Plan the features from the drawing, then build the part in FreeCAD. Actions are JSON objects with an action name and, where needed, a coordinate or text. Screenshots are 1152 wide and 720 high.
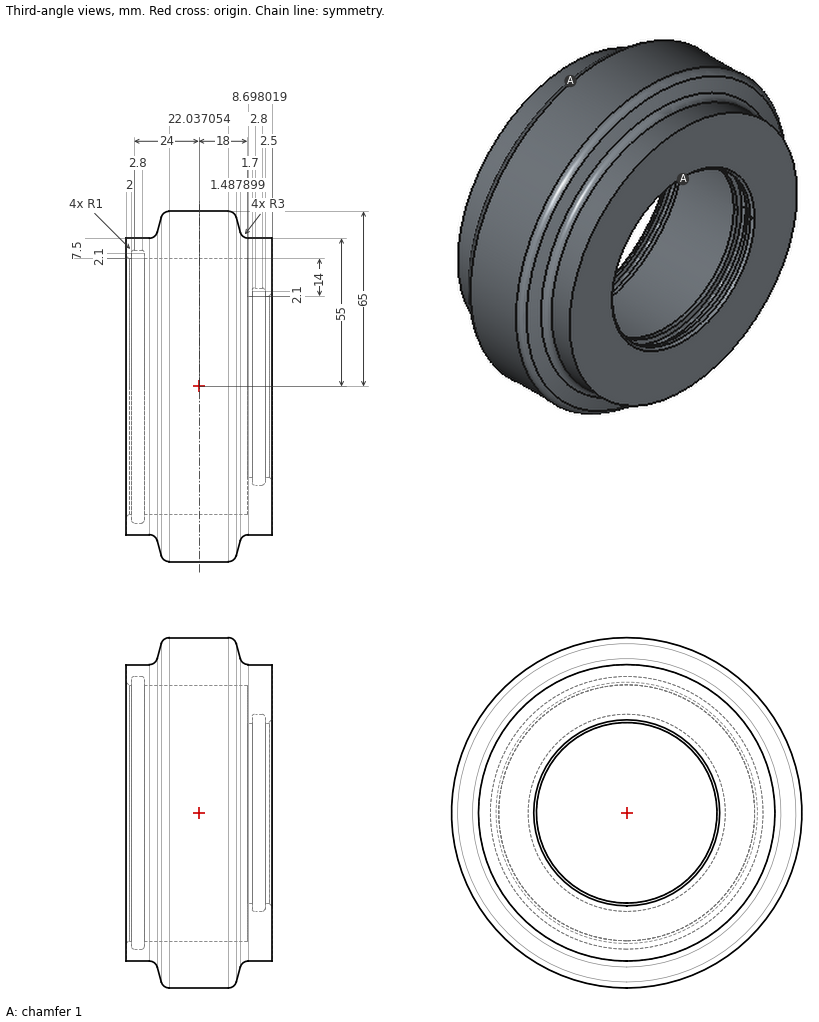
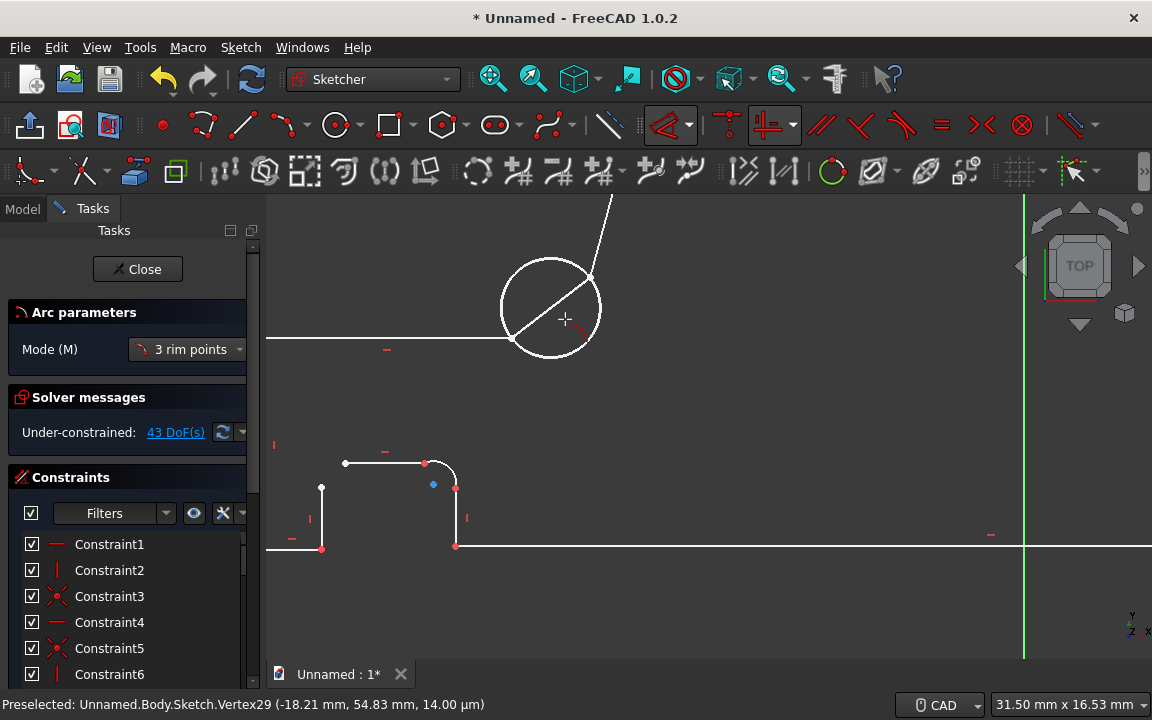
{"action": "left_click", "coordinate": [560, 316]}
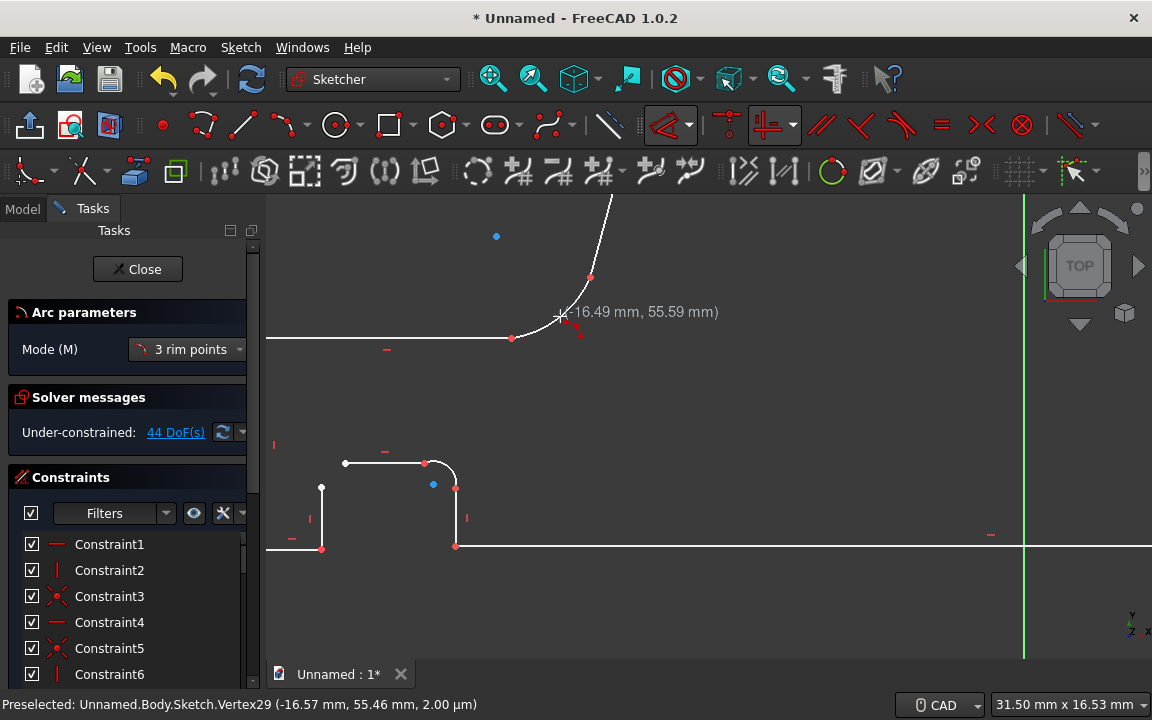
{"action": "left_click", "coordinate": [322, 488]}
{"action": "left_click", "coordinate": [346, 463]}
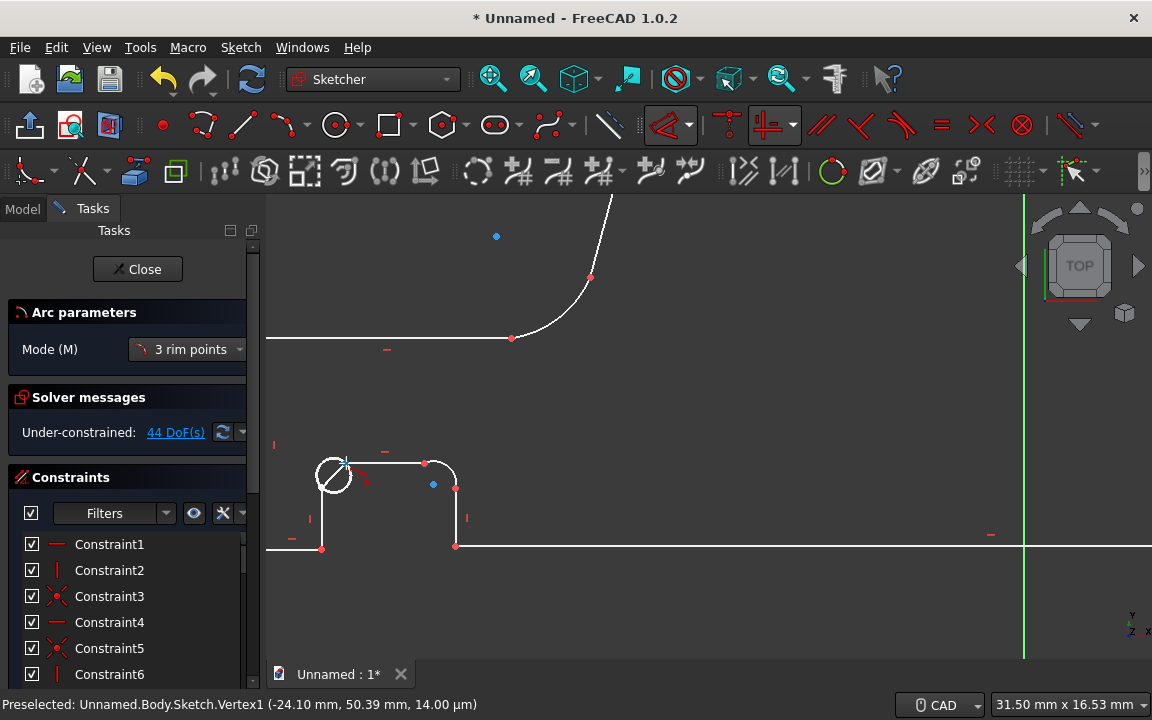
{"action": "scroll", "coordinate": [329, 465], "scroll_direction": "up", "scroll_amount": 4}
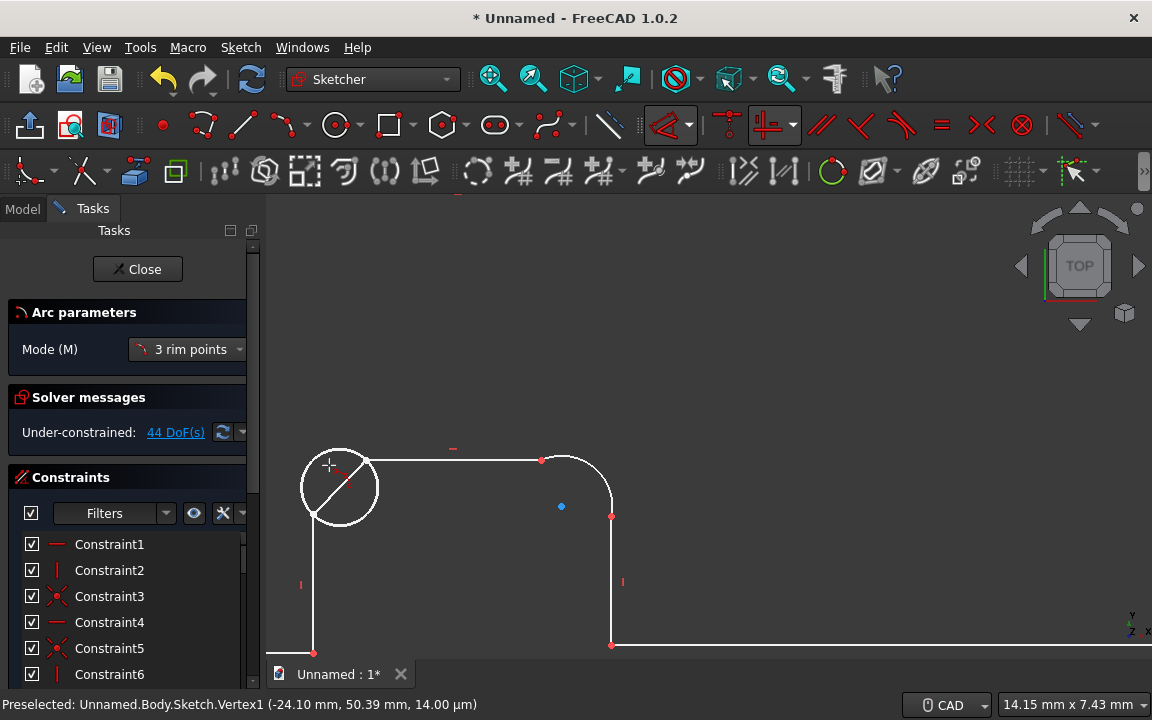
{"action": "left_click", "coordinate": [328, 465]}
{"action": "key", "text": "Escape"}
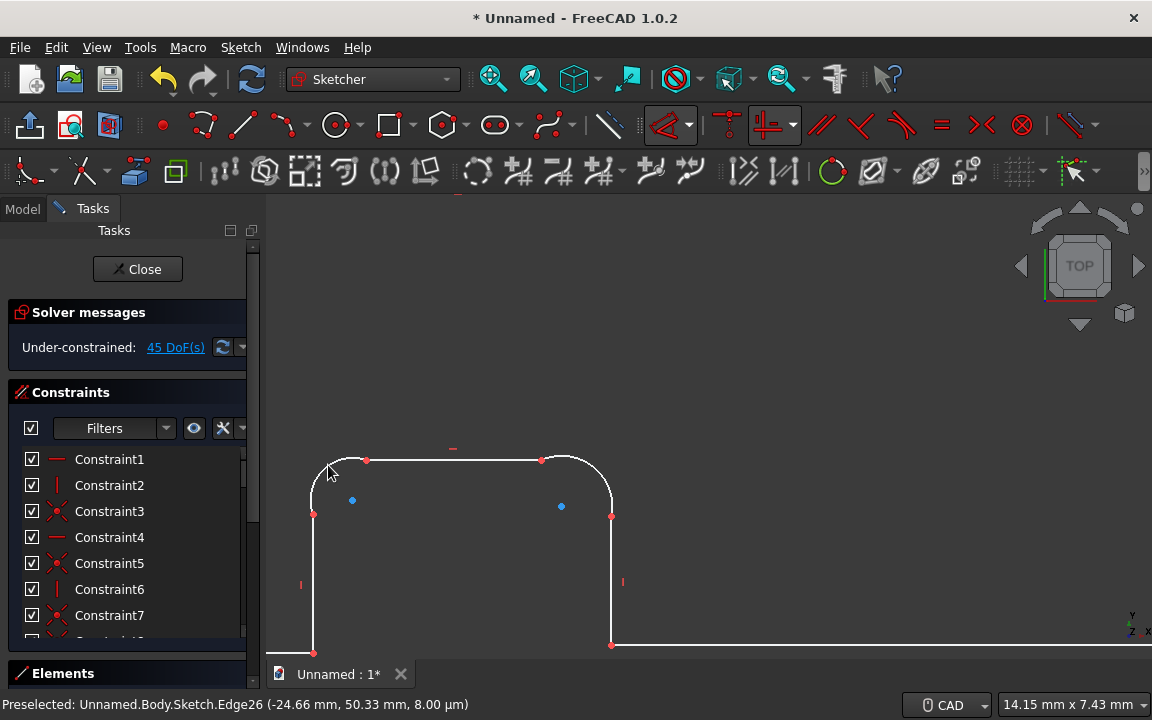
{"action": "scroll", "coordinate": [541, 334], "scroll_direction": "down", "scroll_amount": 13}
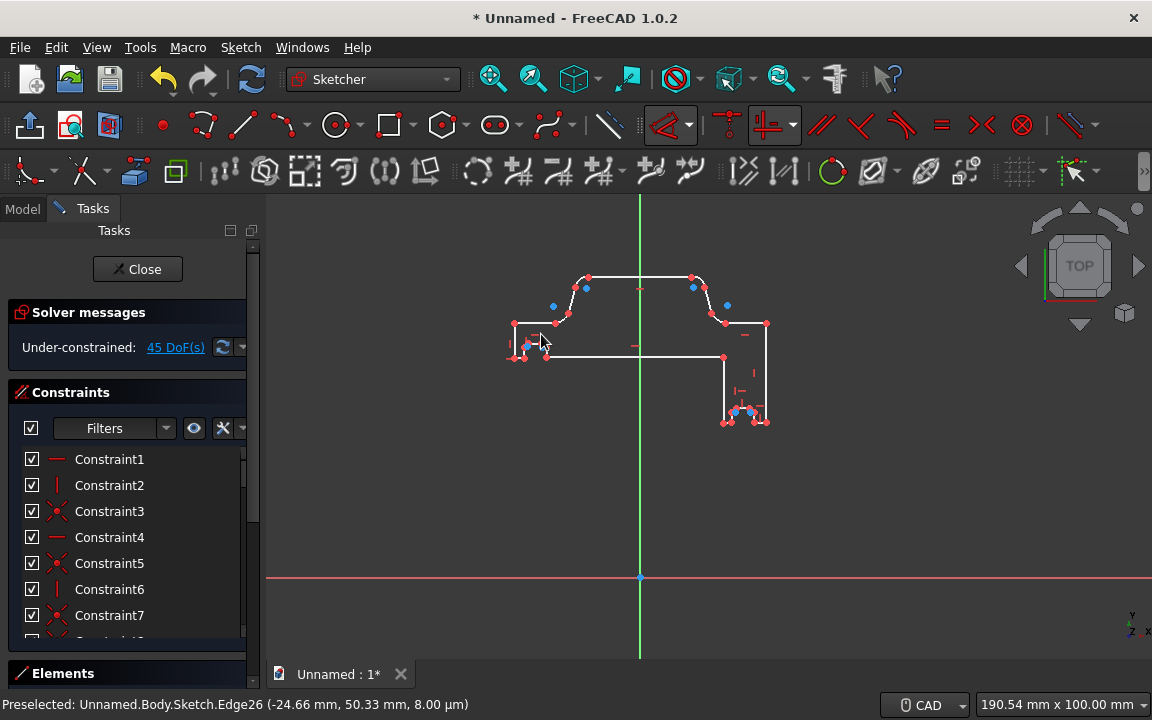
{"action": "scroll", "coordinate": [532, 344], "scroll_direction": "up", "scroll_amount": 7}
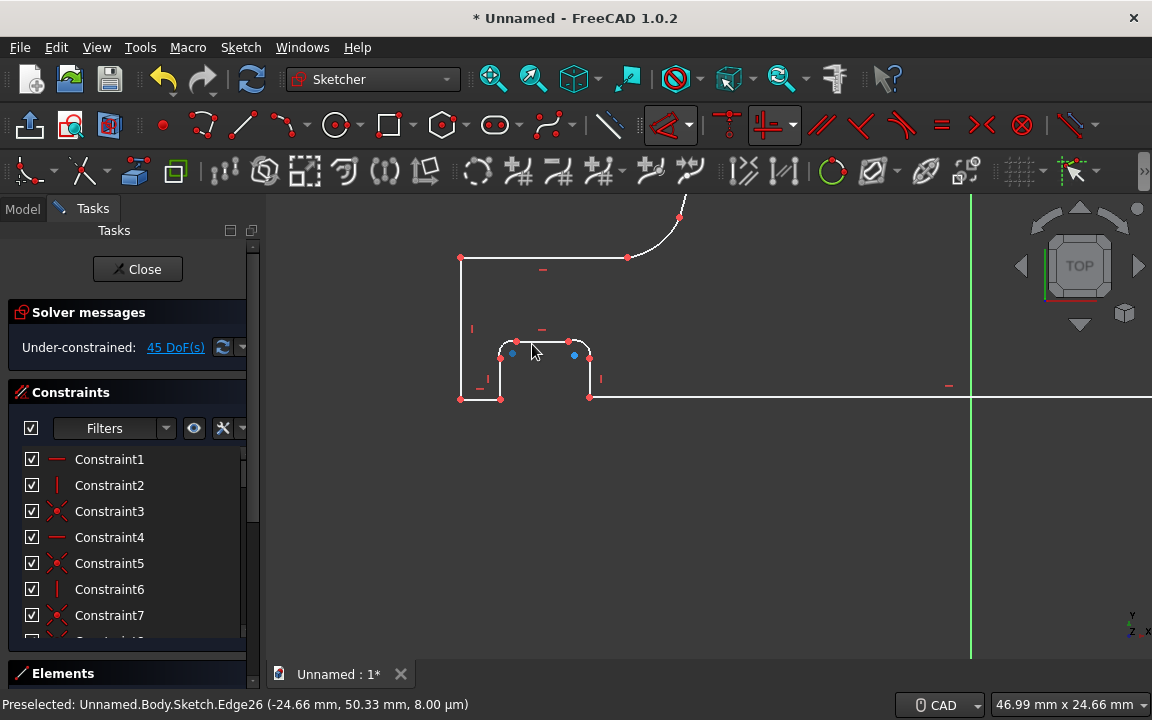
{"action": "left_click", "coordinate": [532, 342]}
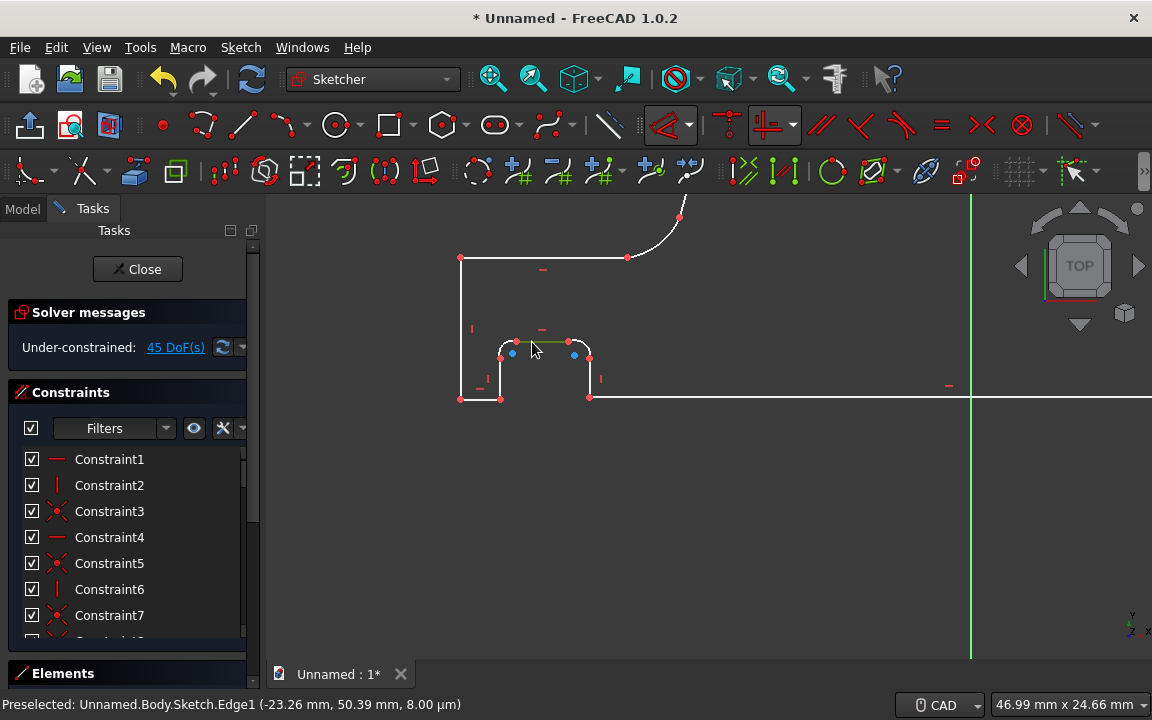
{"action": "scroll", "coordinate": [589, 349], "scroll_direction": "up", "scroll_amount": 2}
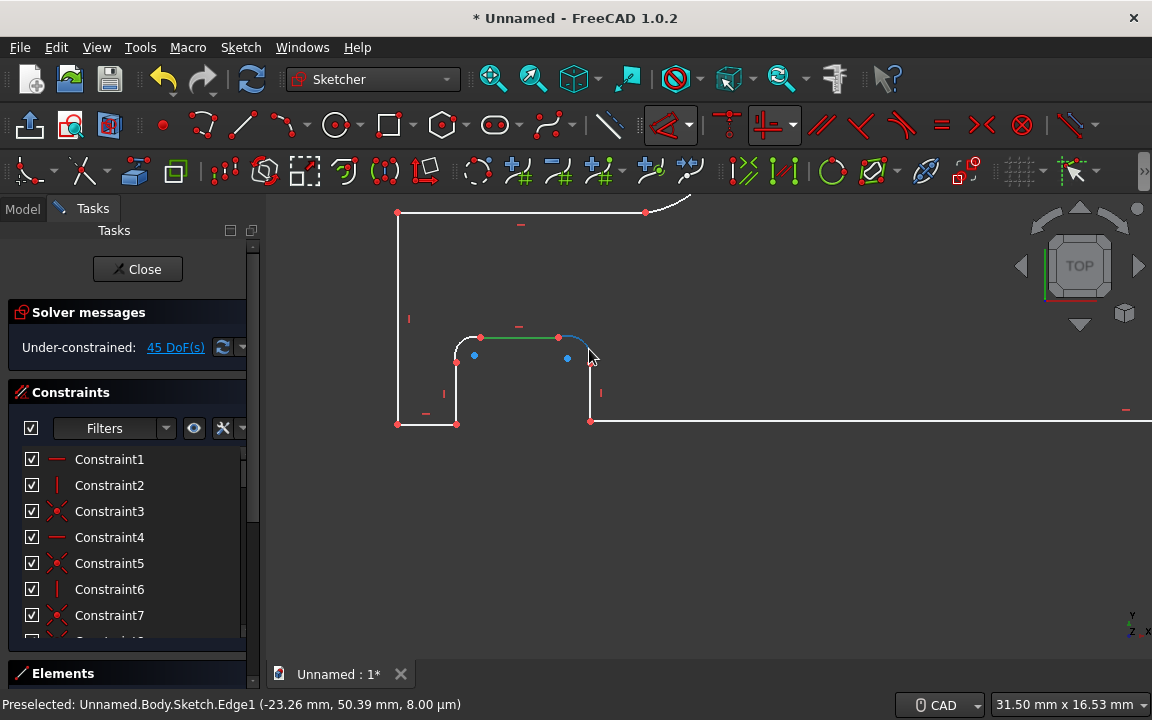
{"action": "left_click", "coordinate": [588, 349]}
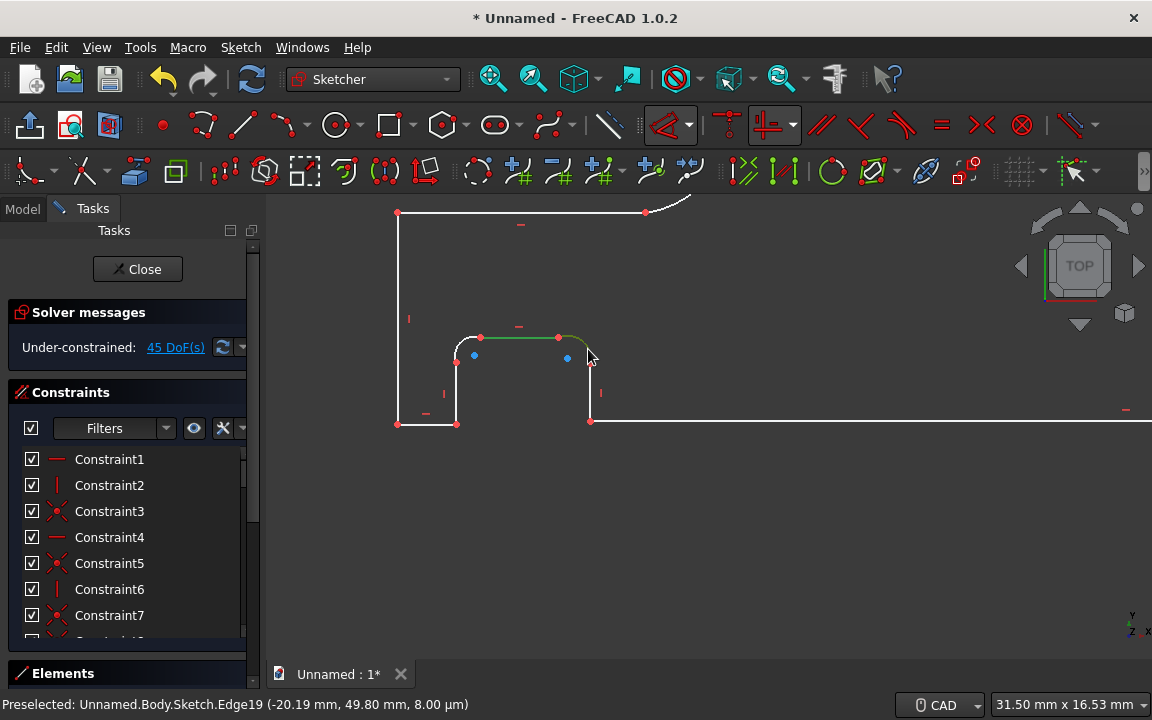
{"action": "left_click", "coordinate": [902, 126]}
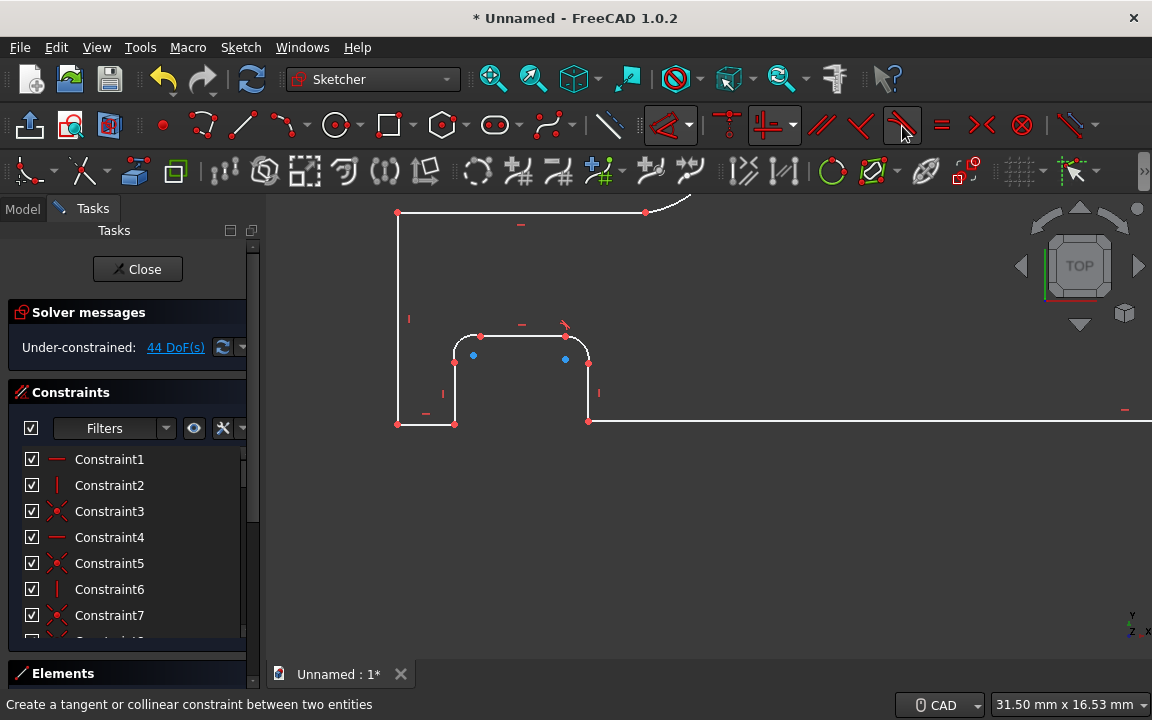
{"action": "left_click", "coordinate": [506, 336]}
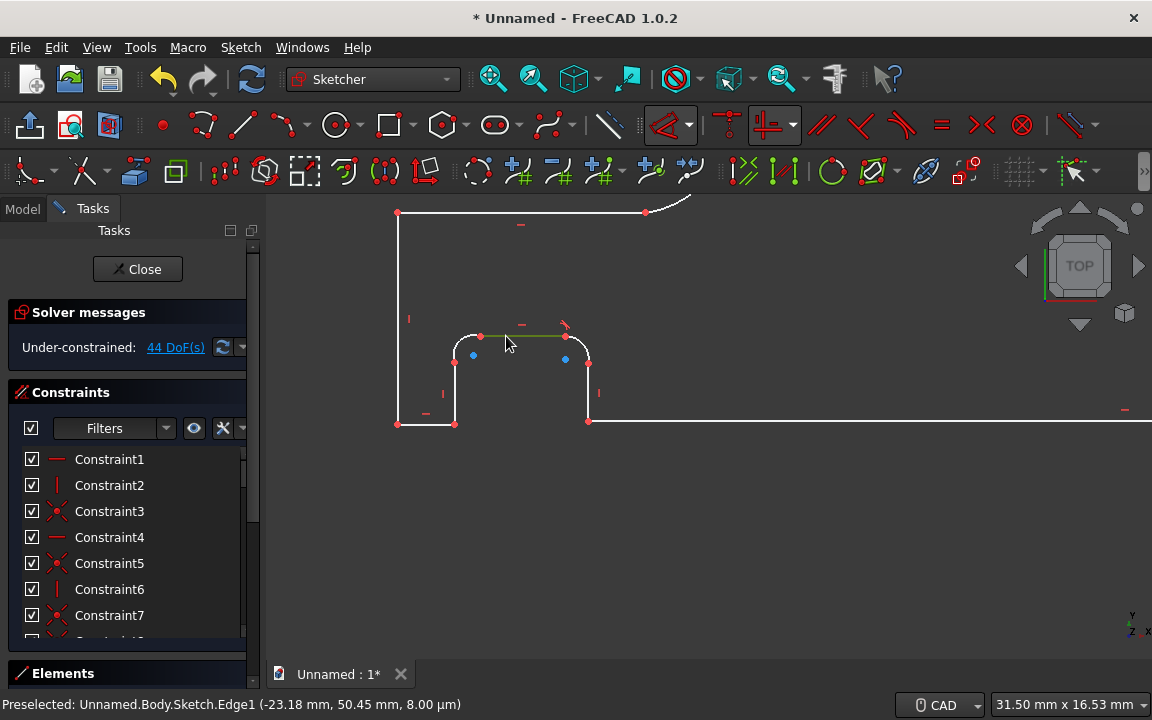
{"action": "left_click", "coordinate": [467, 336]}